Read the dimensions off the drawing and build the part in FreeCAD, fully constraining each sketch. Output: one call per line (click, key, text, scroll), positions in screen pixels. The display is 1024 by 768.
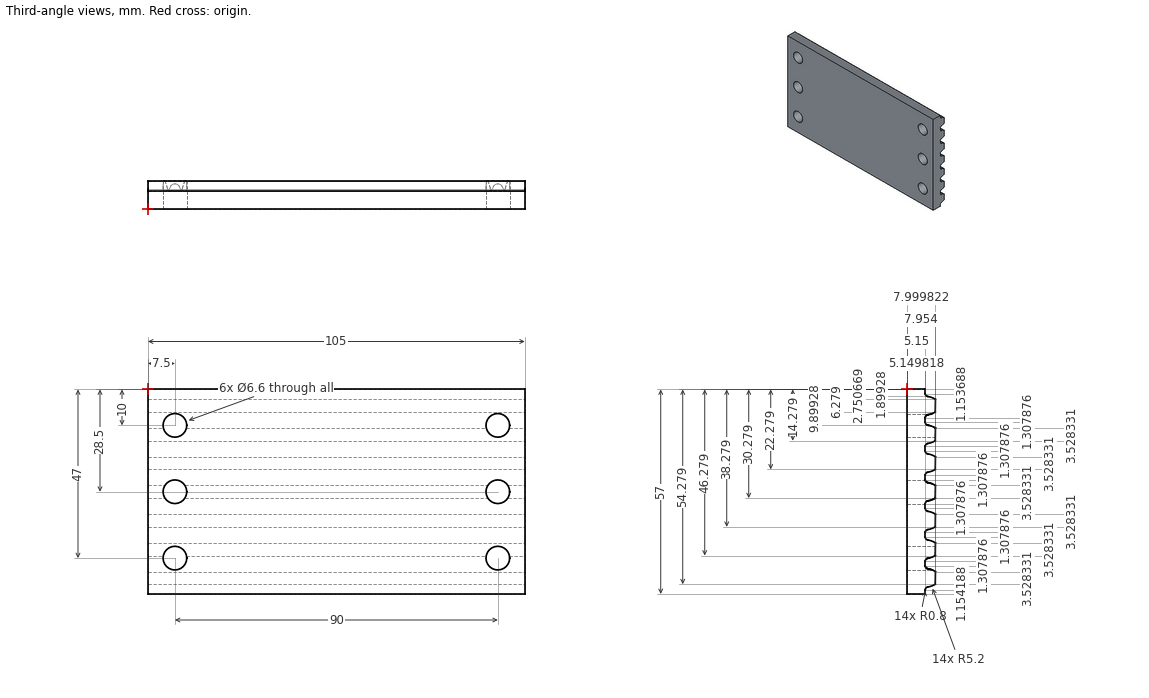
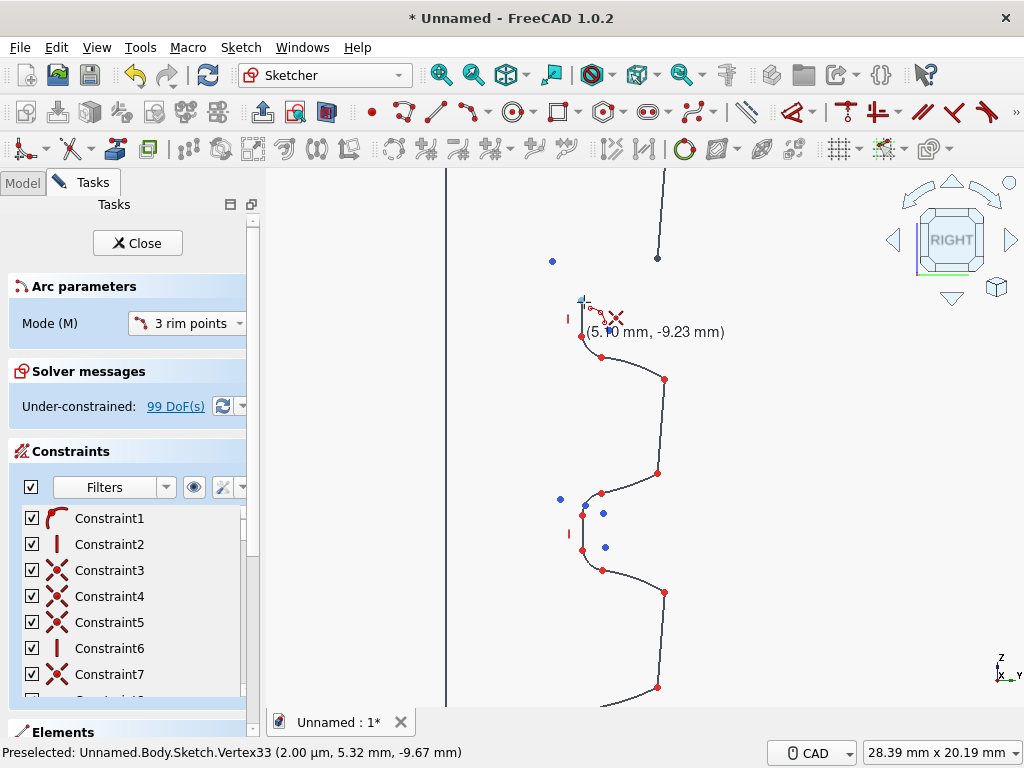
click(582, 301)
click(602, 279)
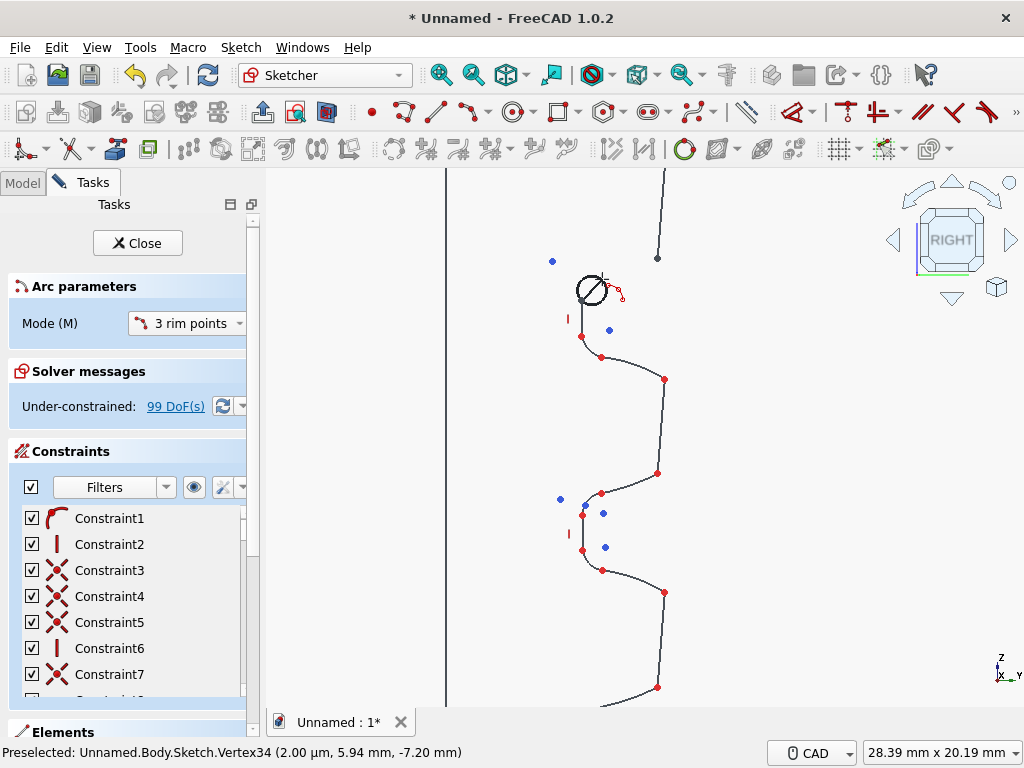
scroll(588, 286, up, 6)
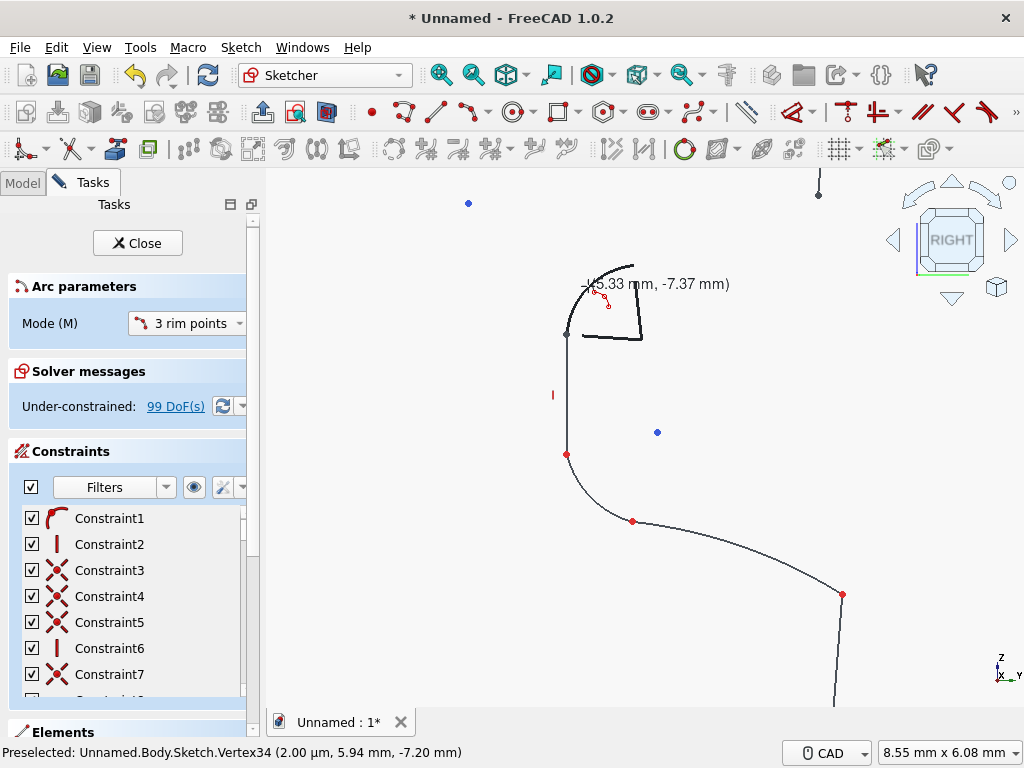
click(589, 284)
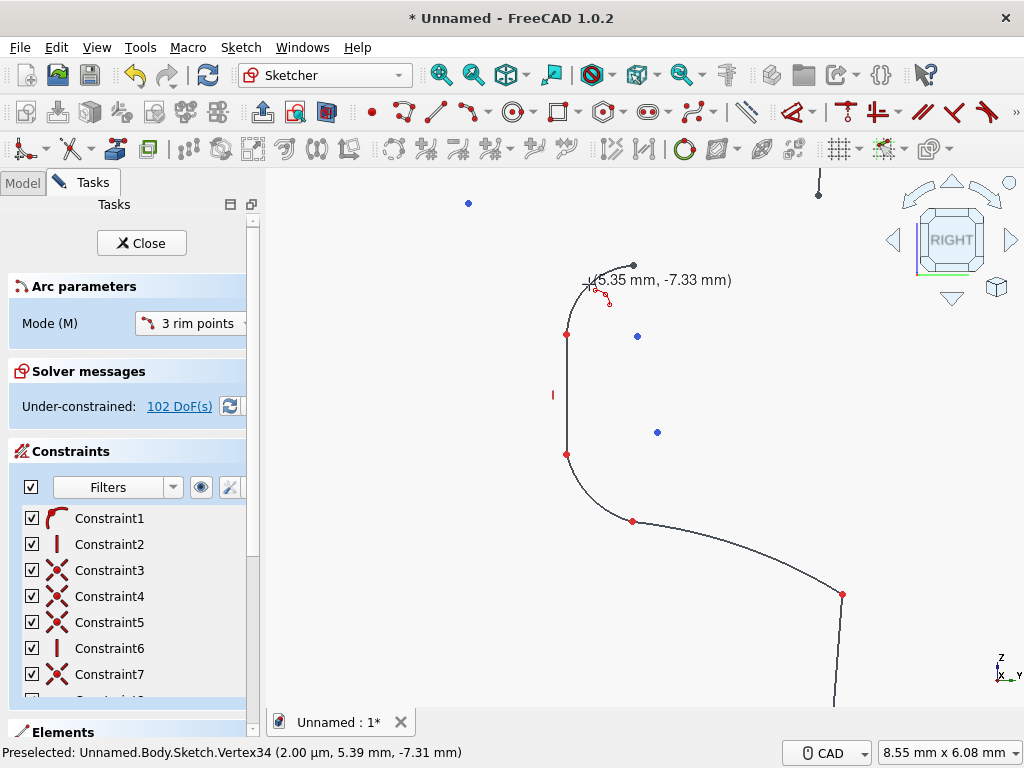
scroll(585, 299, down, 13)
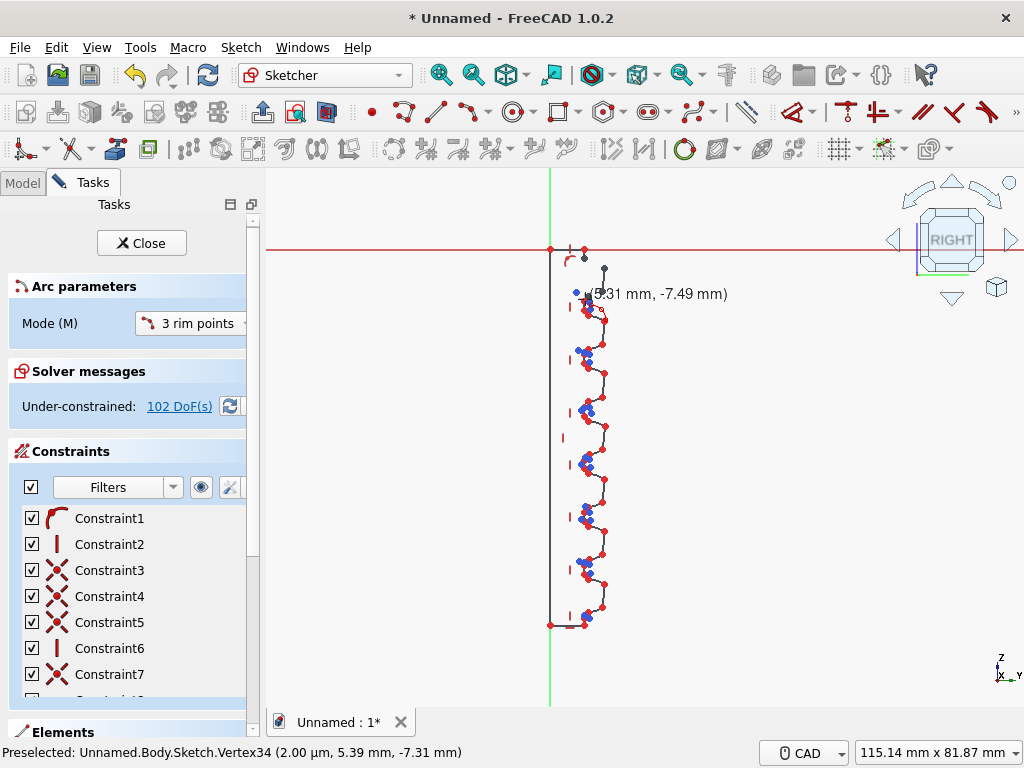
scroll(589, 296, up, 6)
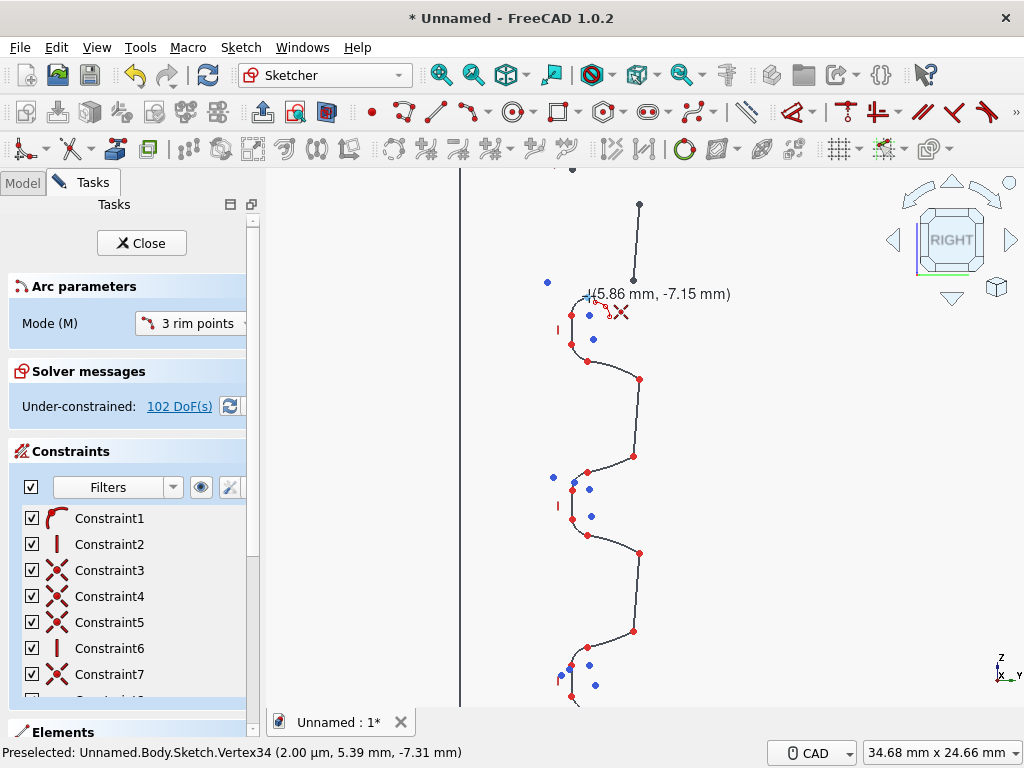
click(588, 298)
click(634, 281)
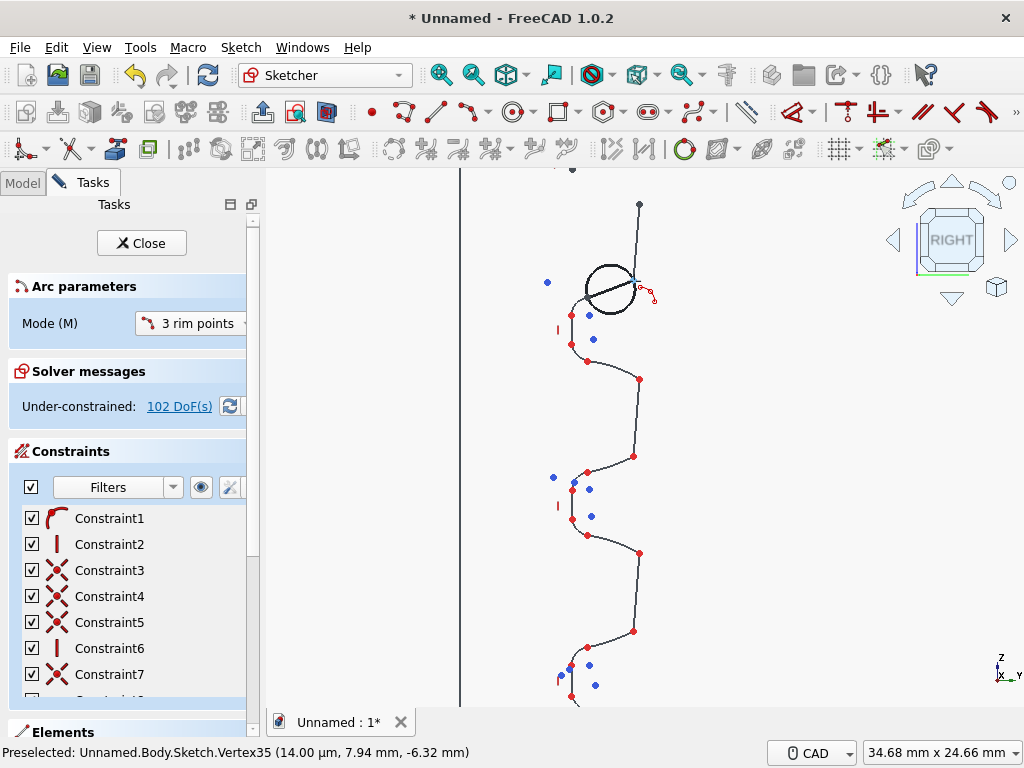
scroll(612, 291, up, 9)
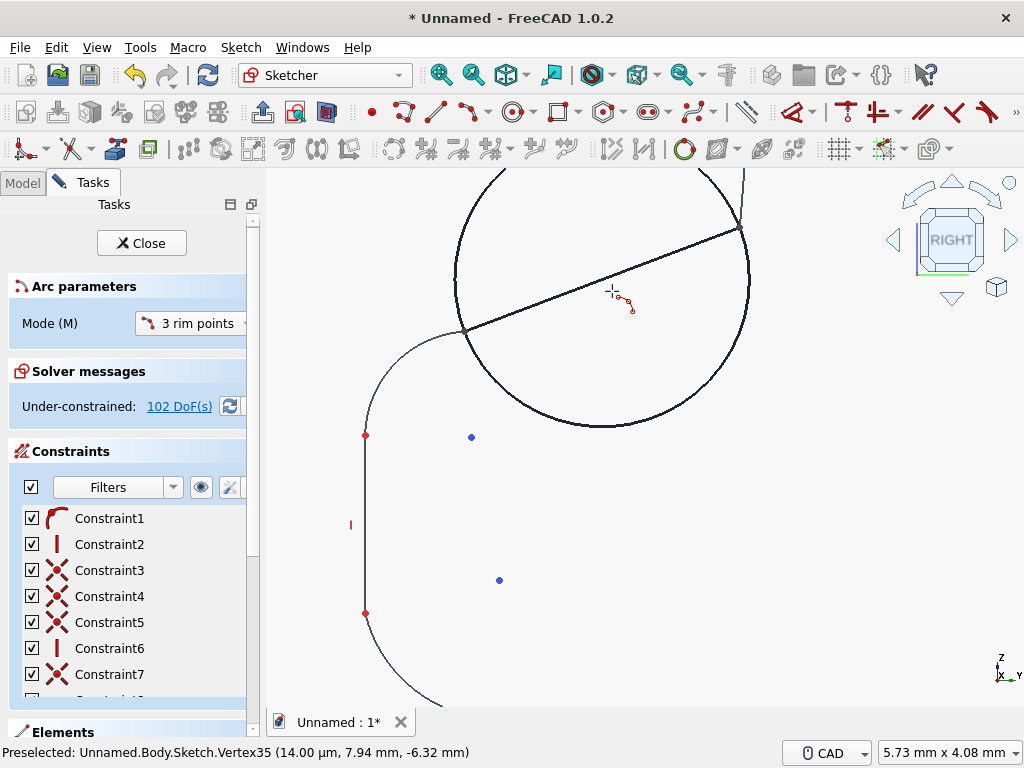
click(608, 289)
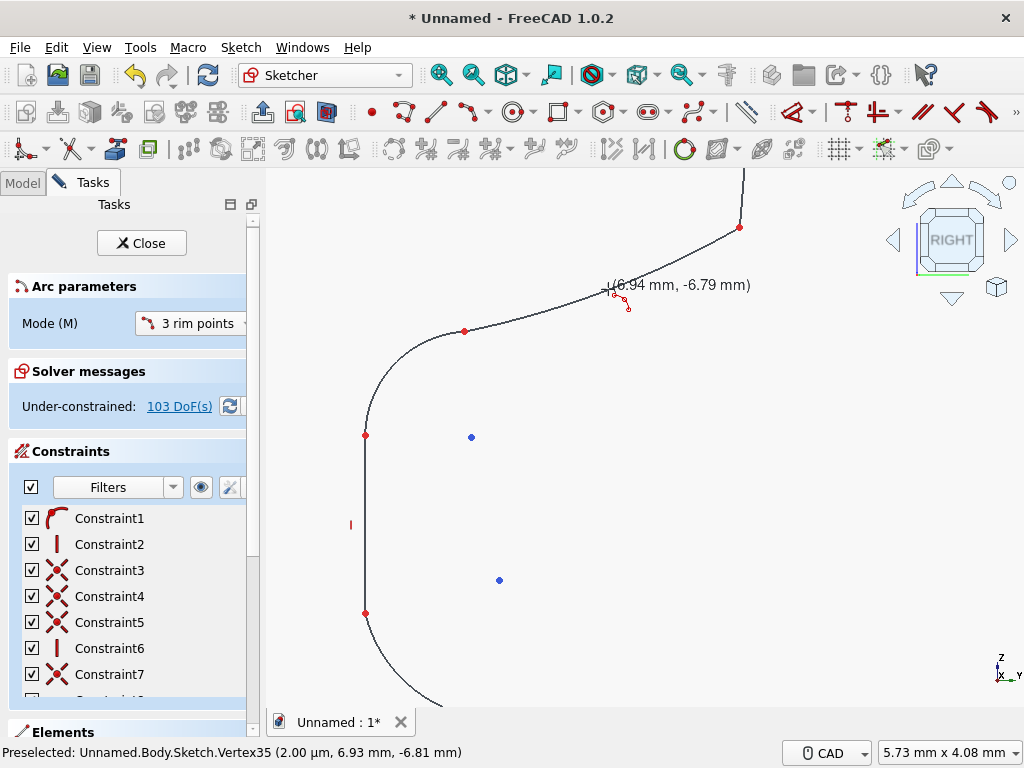
scroll(595, 295, down, 15)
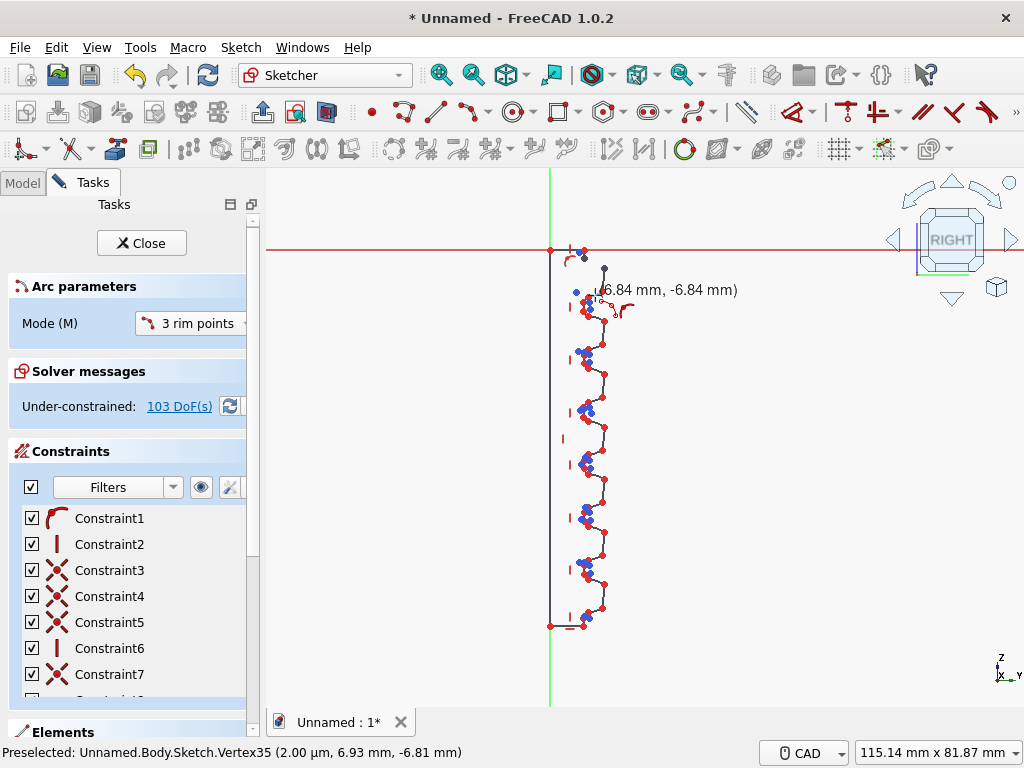
scroll(603, 268, up, 2)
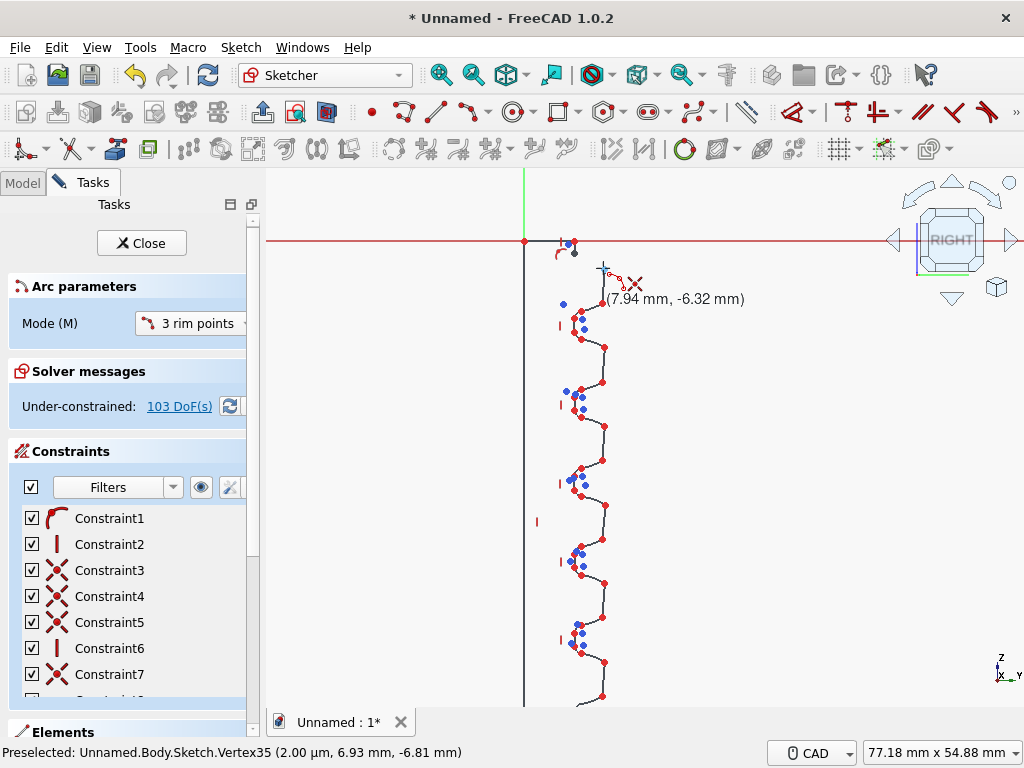
click(605, 269)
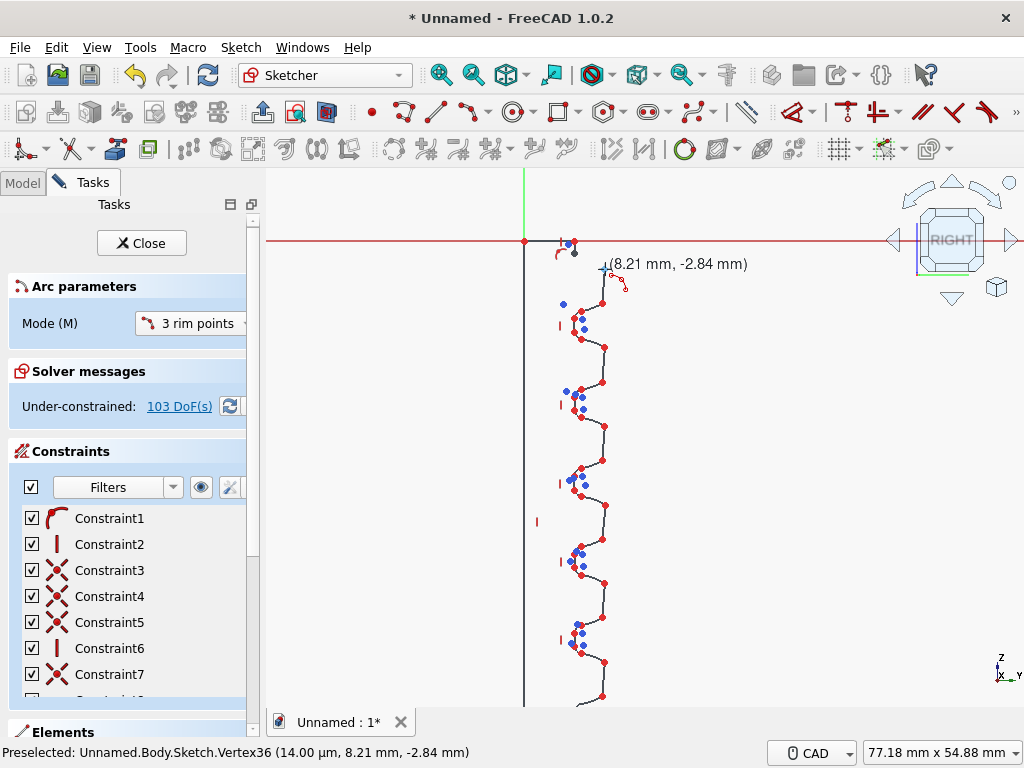
scroll(582, 261, up, 5)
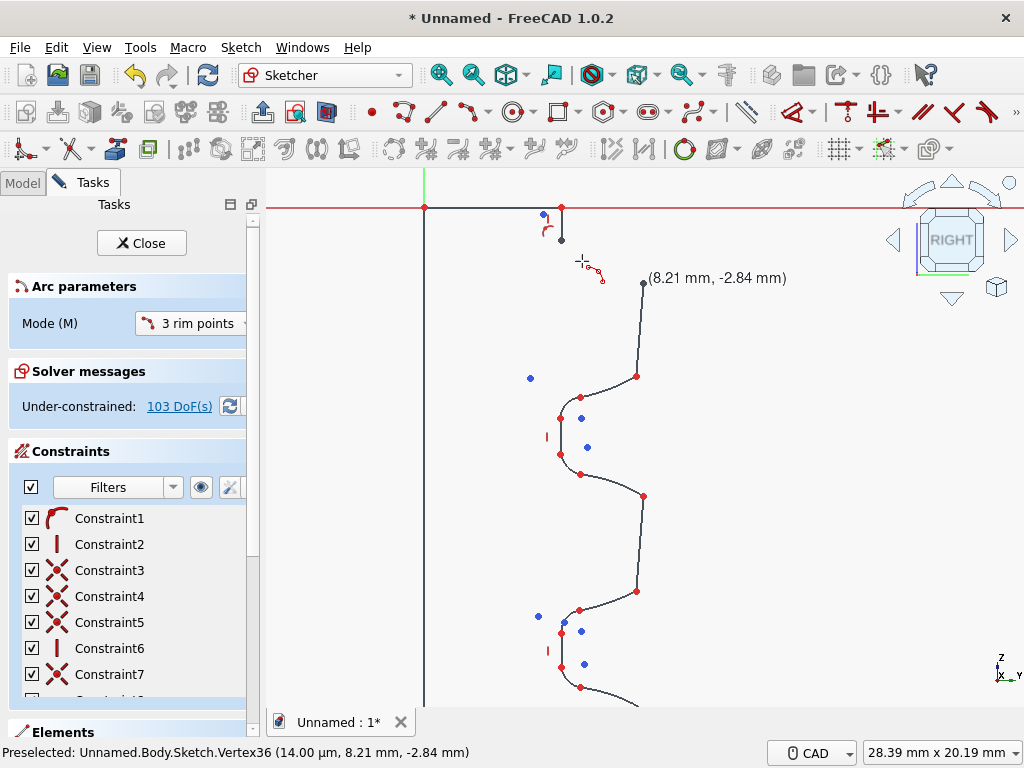
click(580, 260)